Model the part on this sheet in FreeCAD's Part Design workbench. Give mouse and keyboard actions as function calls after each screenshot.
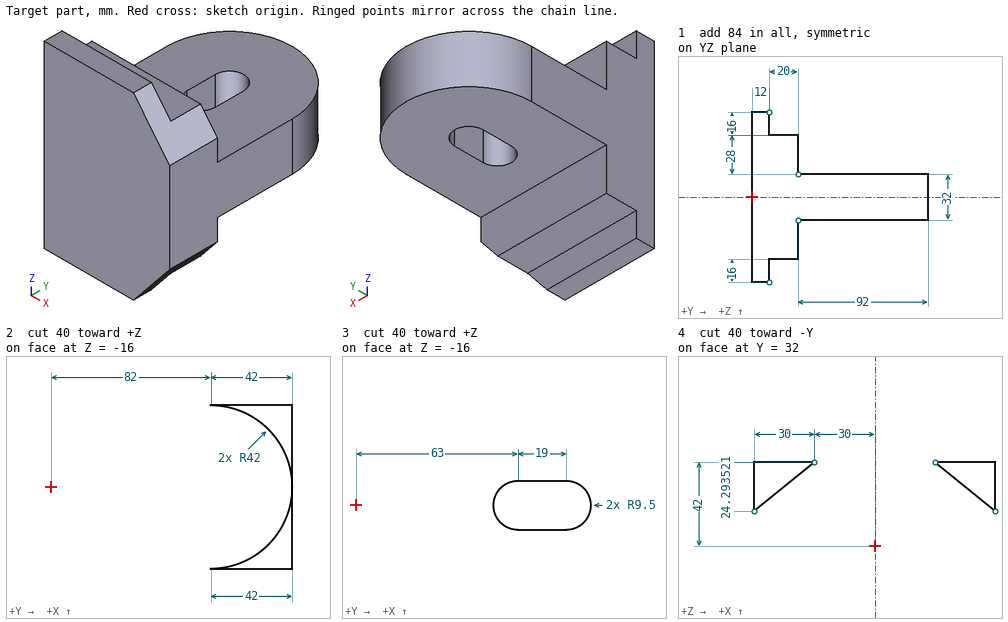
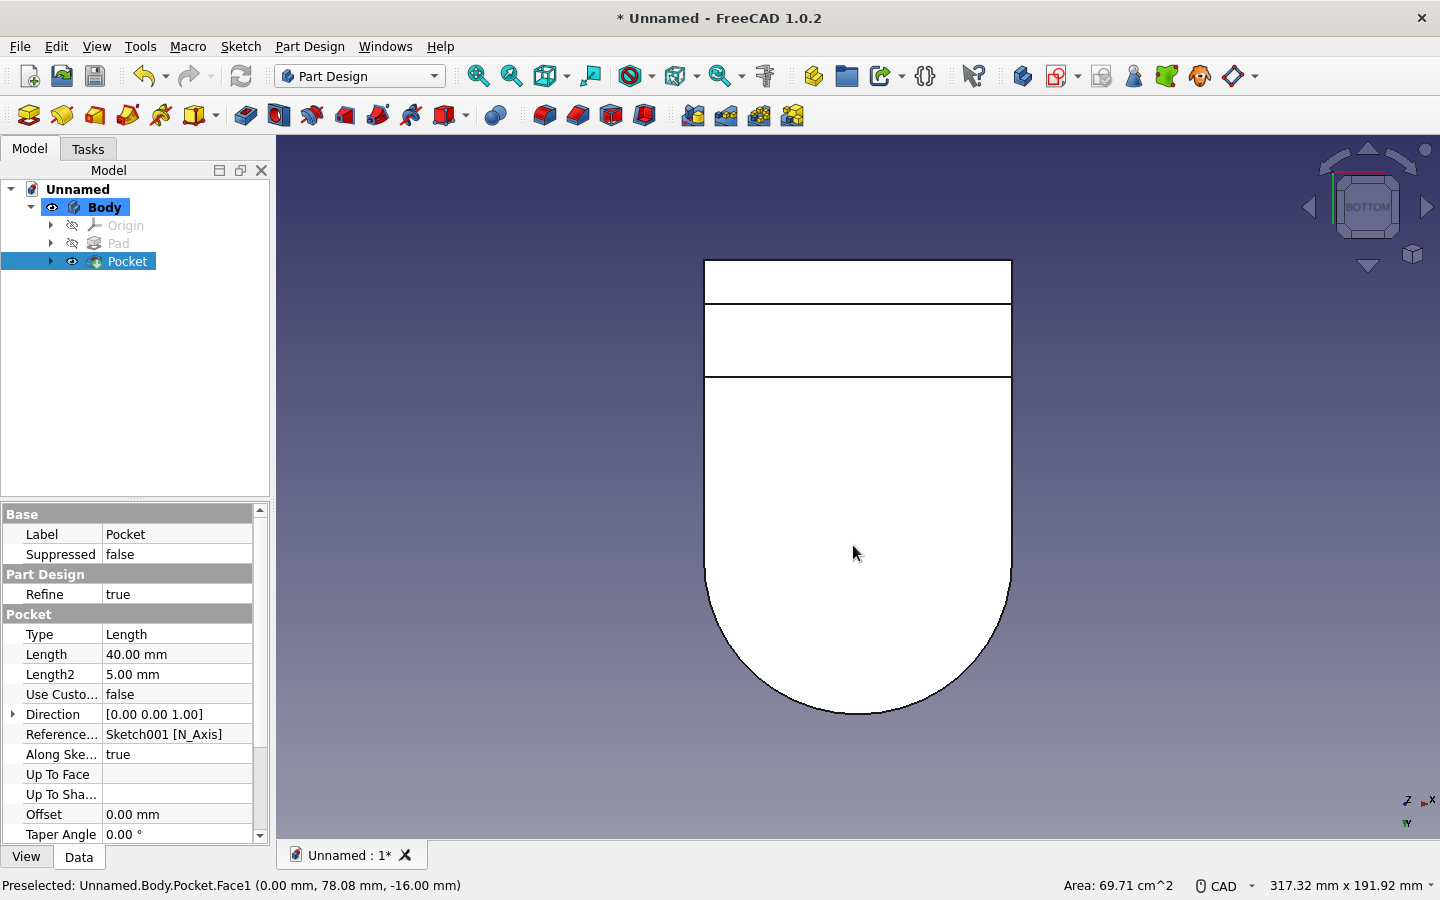
click(1056, 76)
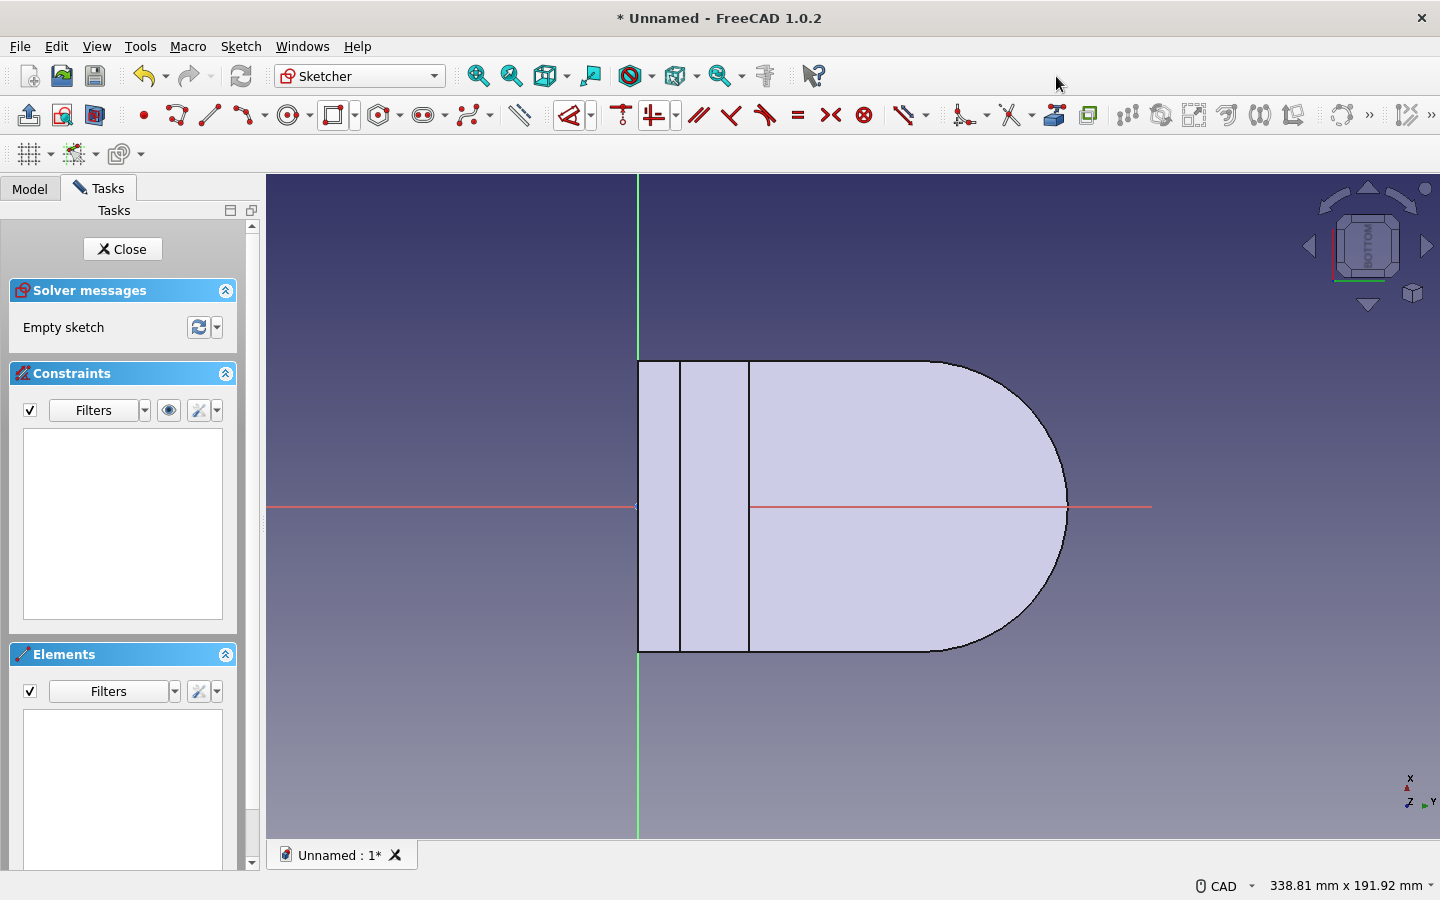
scroll(807, 506, up, 4)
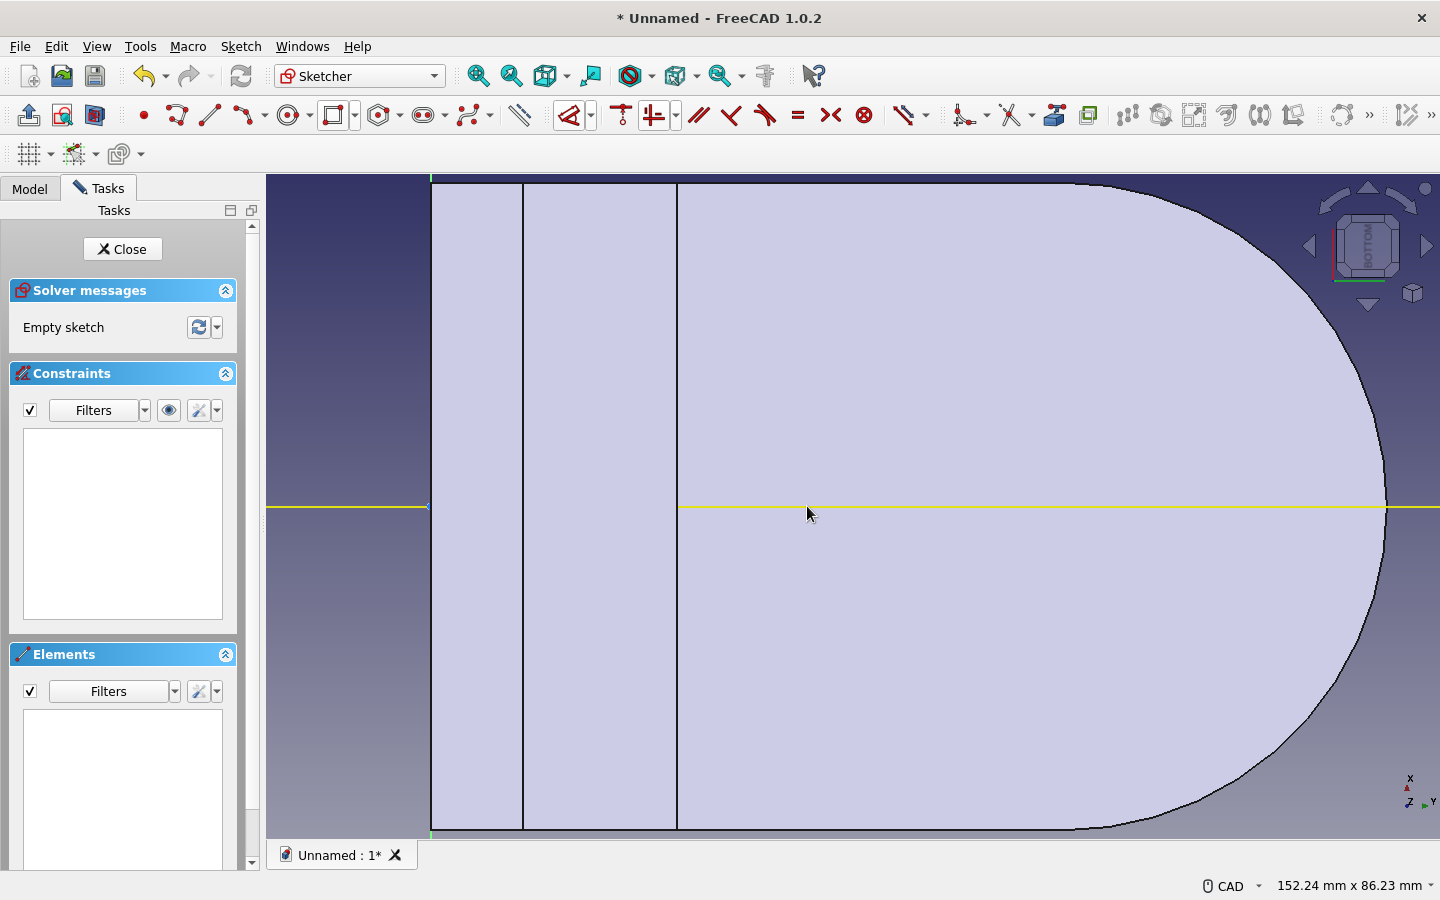
key(g)
key(s)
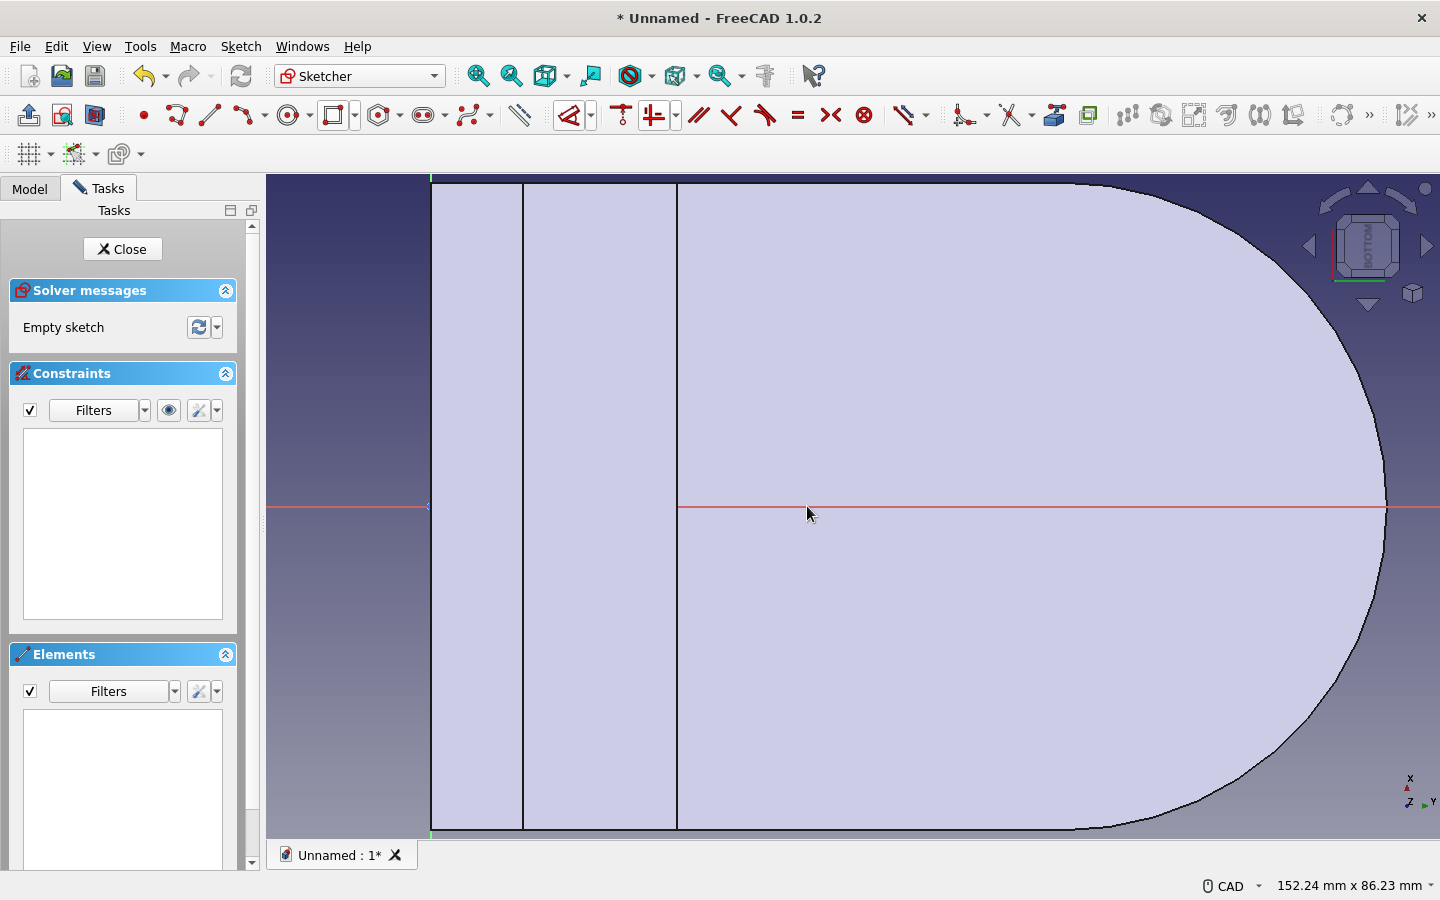
click(917, 506)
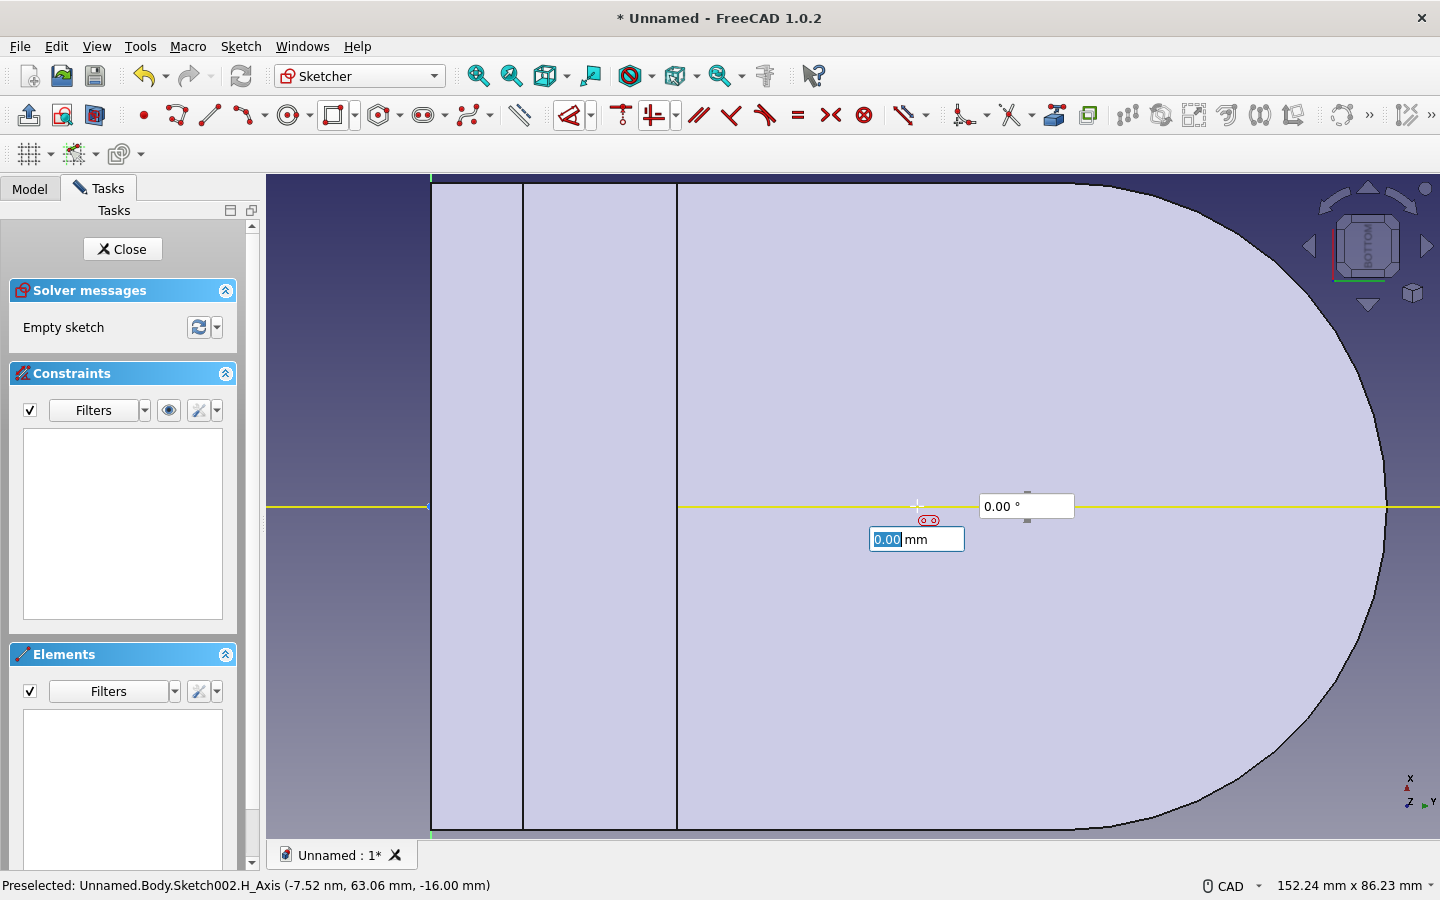
click(1063, 497)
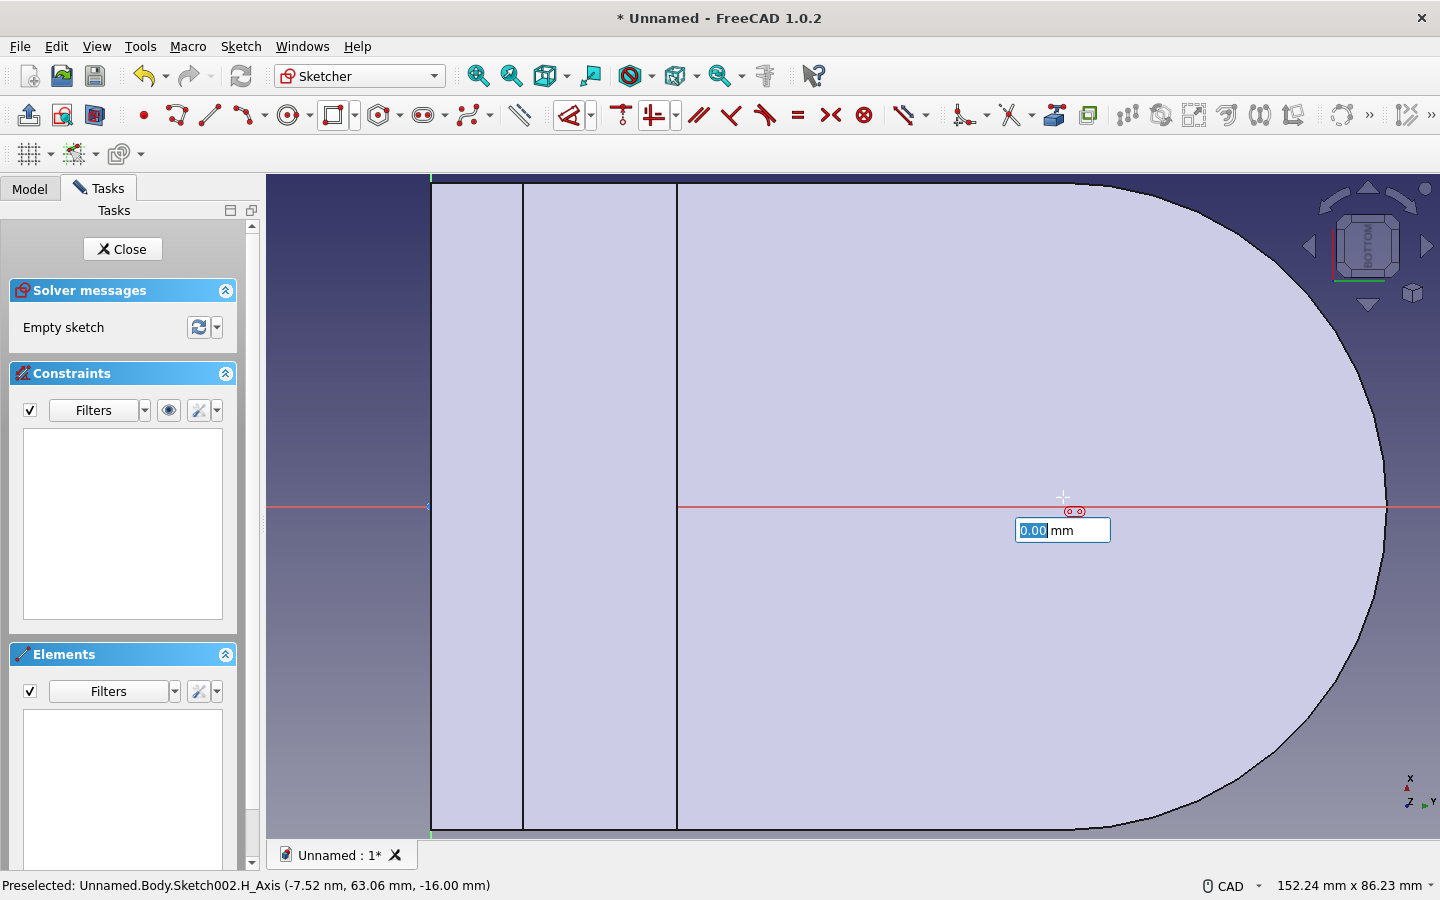
click(990, 580)
key(Escape)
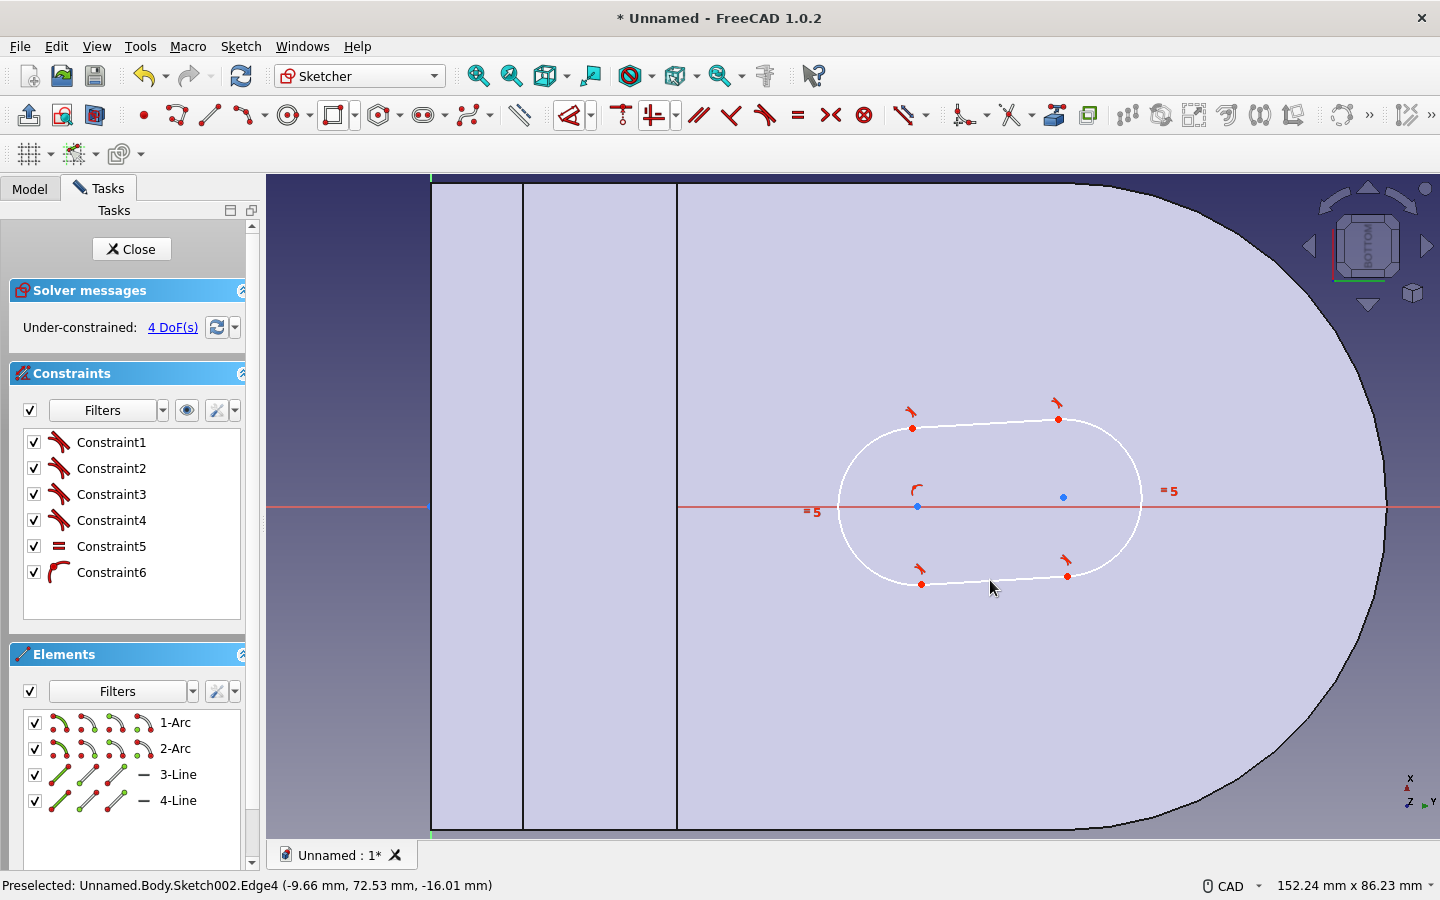
click(956, 425)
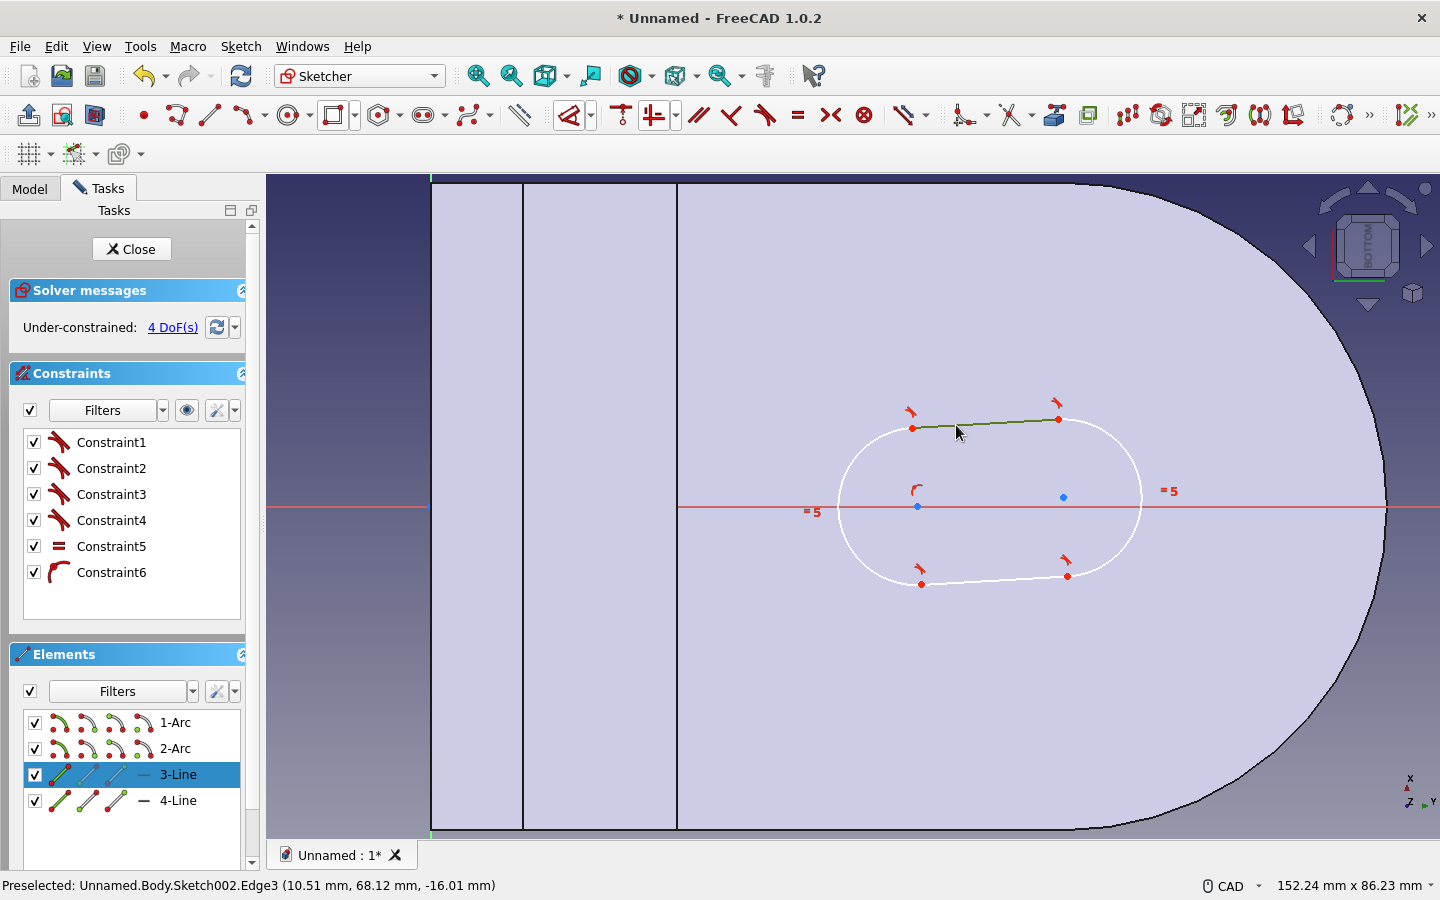
key(h)